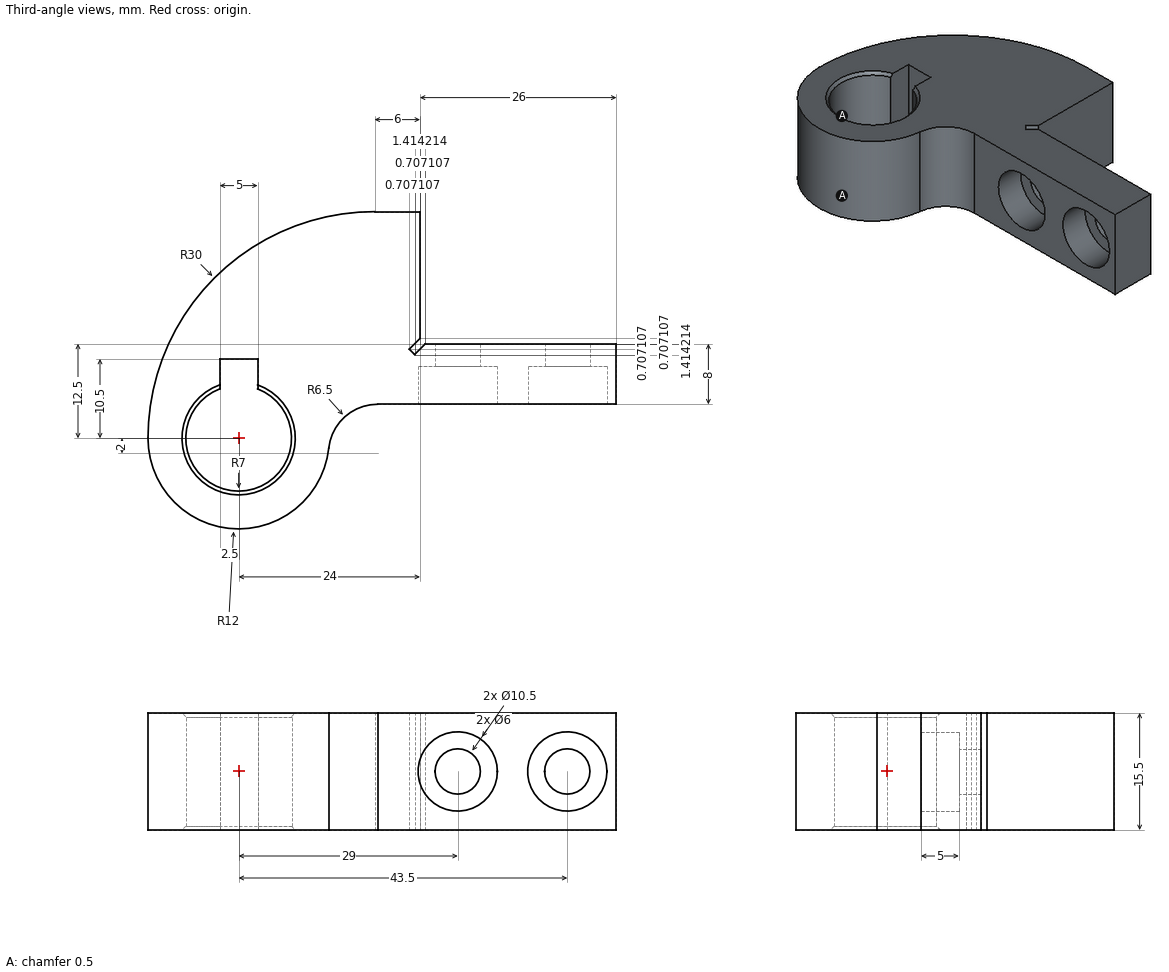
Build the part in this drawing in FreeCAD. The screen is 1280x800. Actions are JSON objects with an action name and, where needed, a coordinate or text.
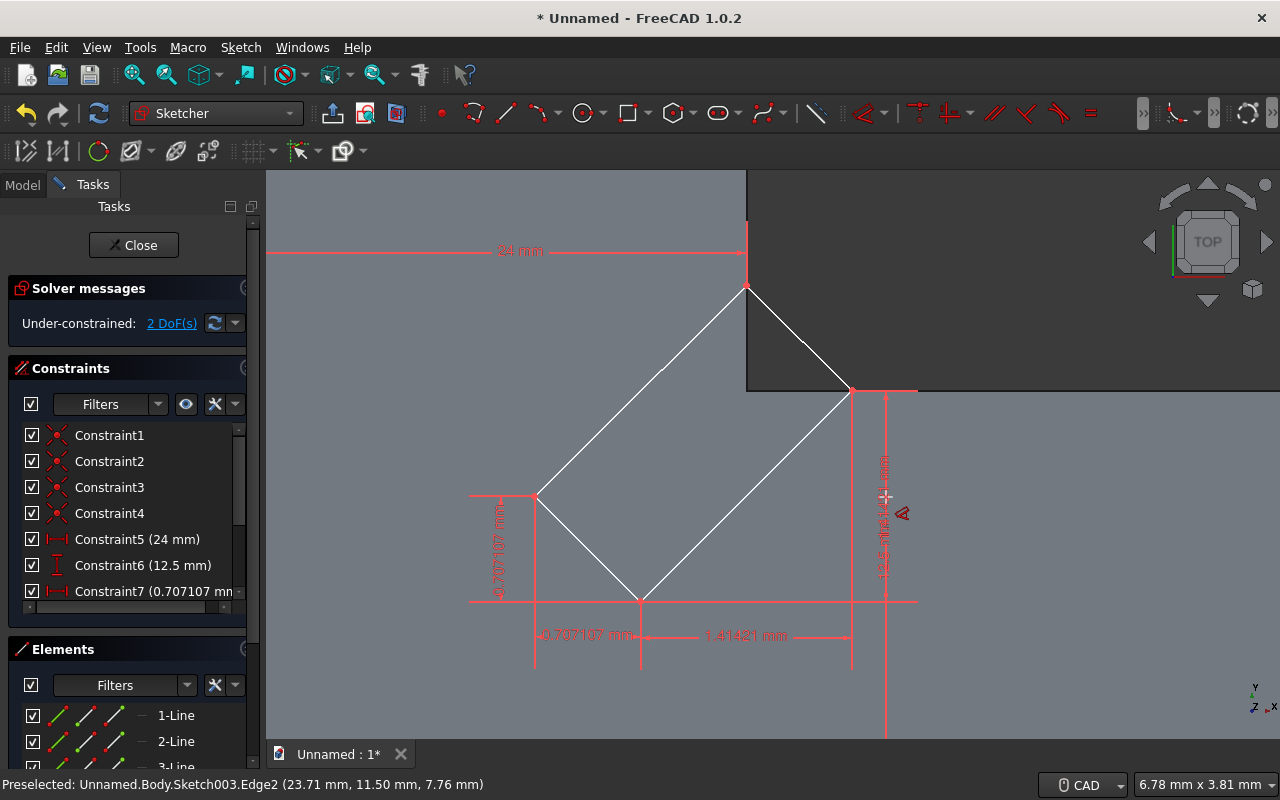
{"action": "left_click", "coordinate": [820, 359]}
{"action": "left_click", "coordinate": [799, 252]}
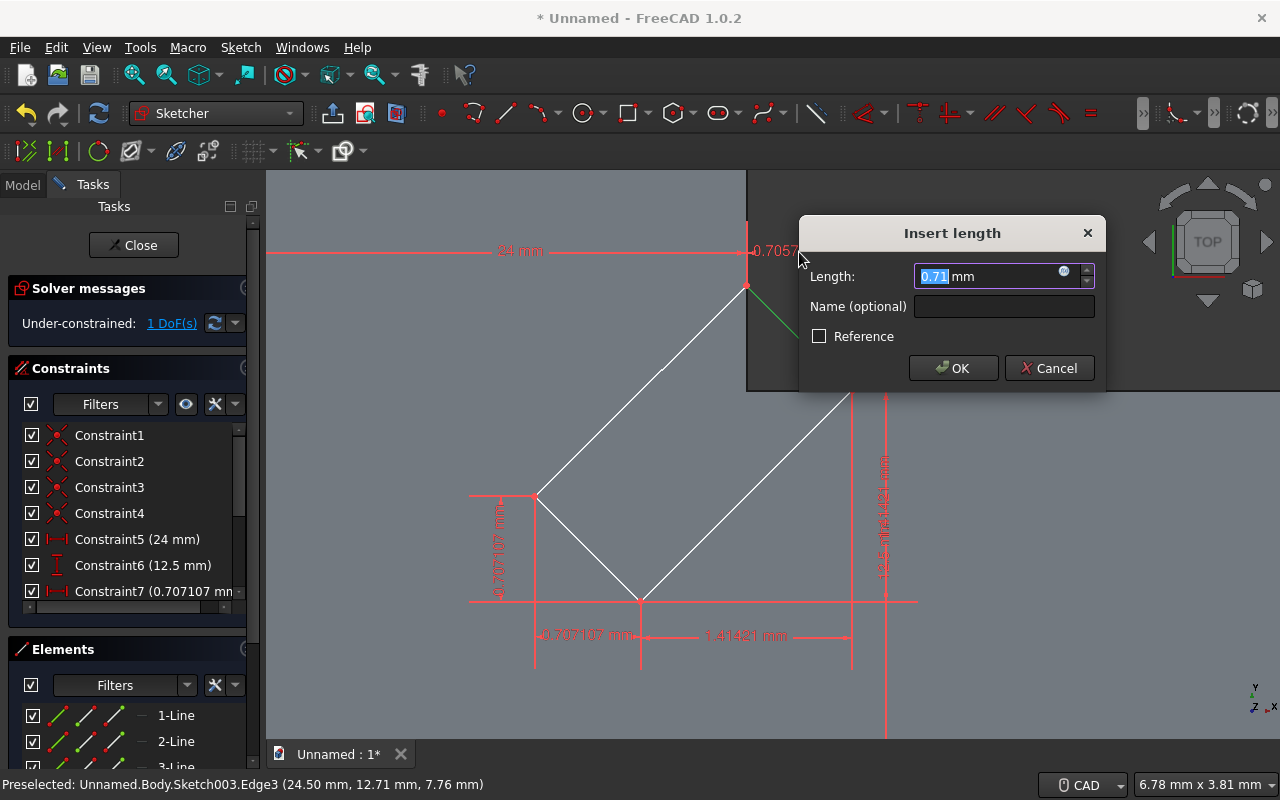
{"action": "type", "text": "0.707107"}
{"action": "key", "text": "Return"}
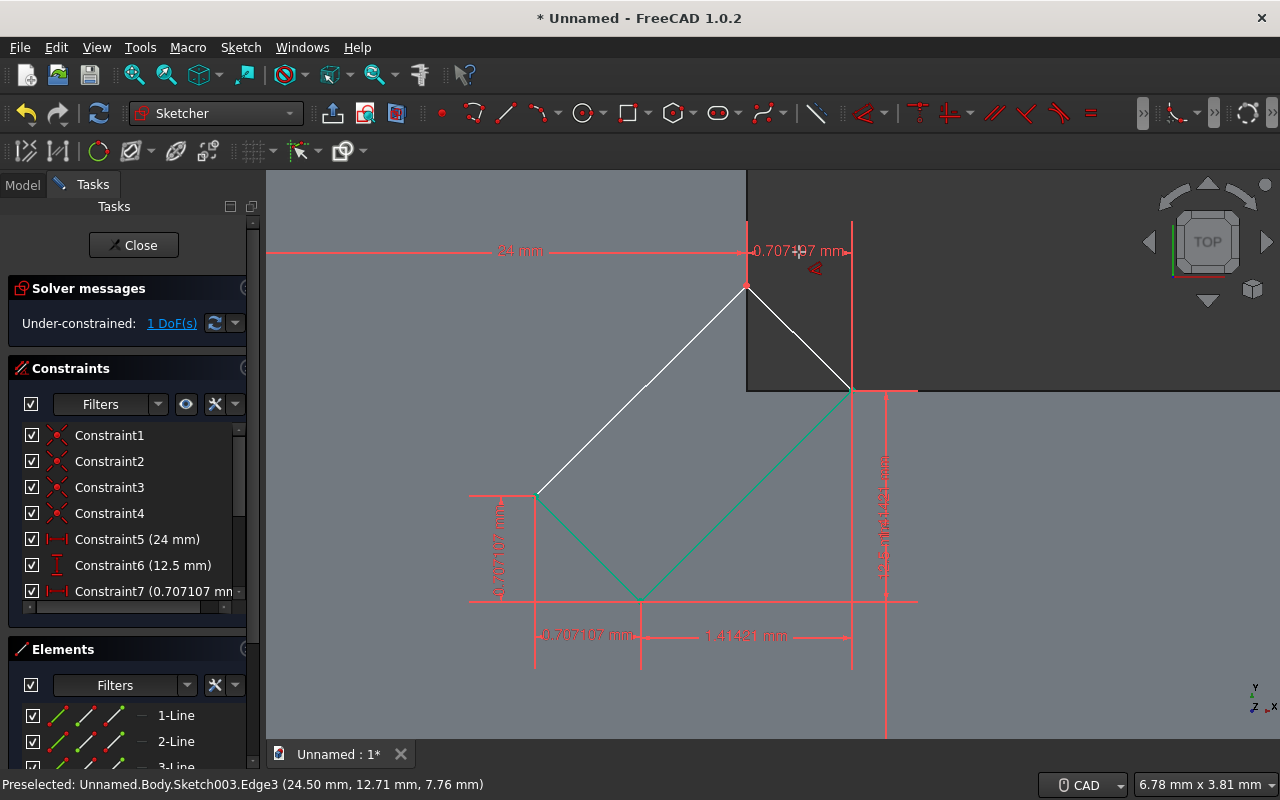
{"action": "left_click", "coordinate": [820, 359]}
{"action": "left_click", "coordinate": [886, 338]}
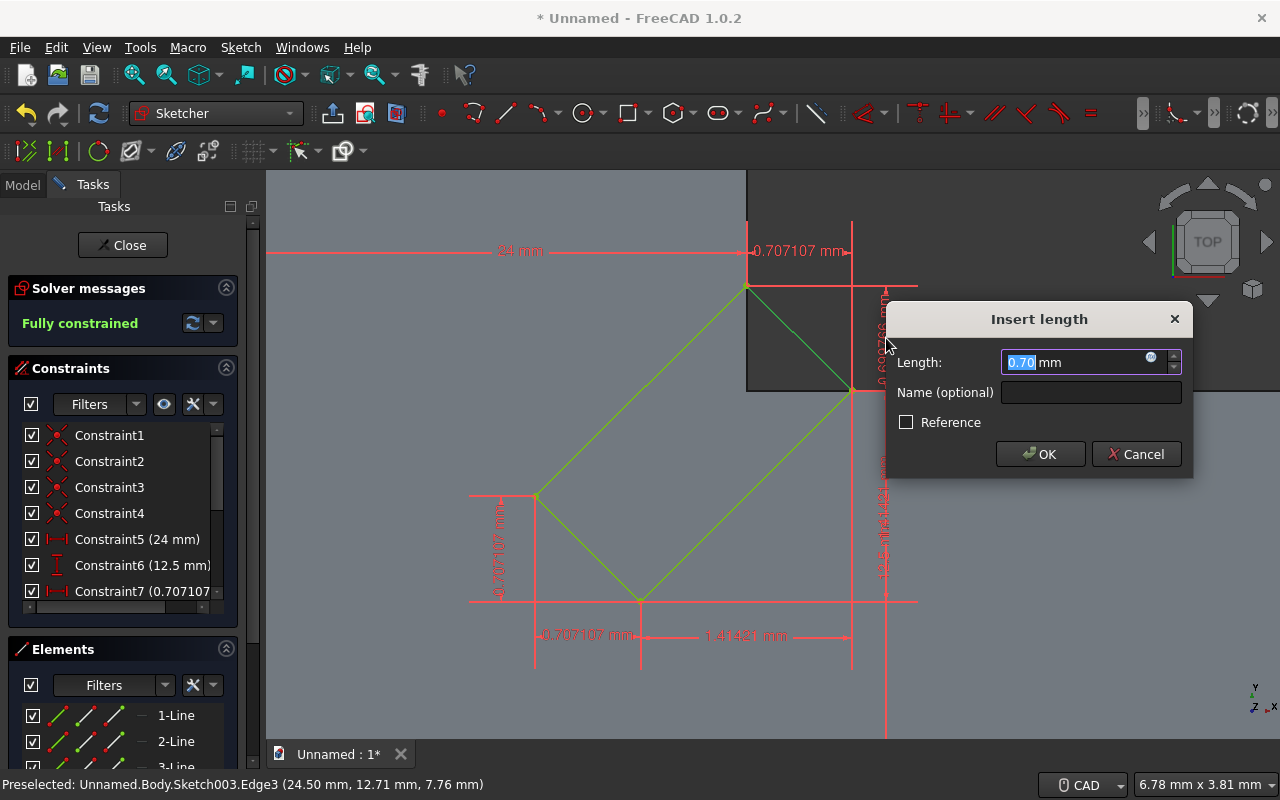
{"action": "type", "text": "0.707107"}
{"action": "key", "text": "Return"}
{"action": "key", "text": "Escape"}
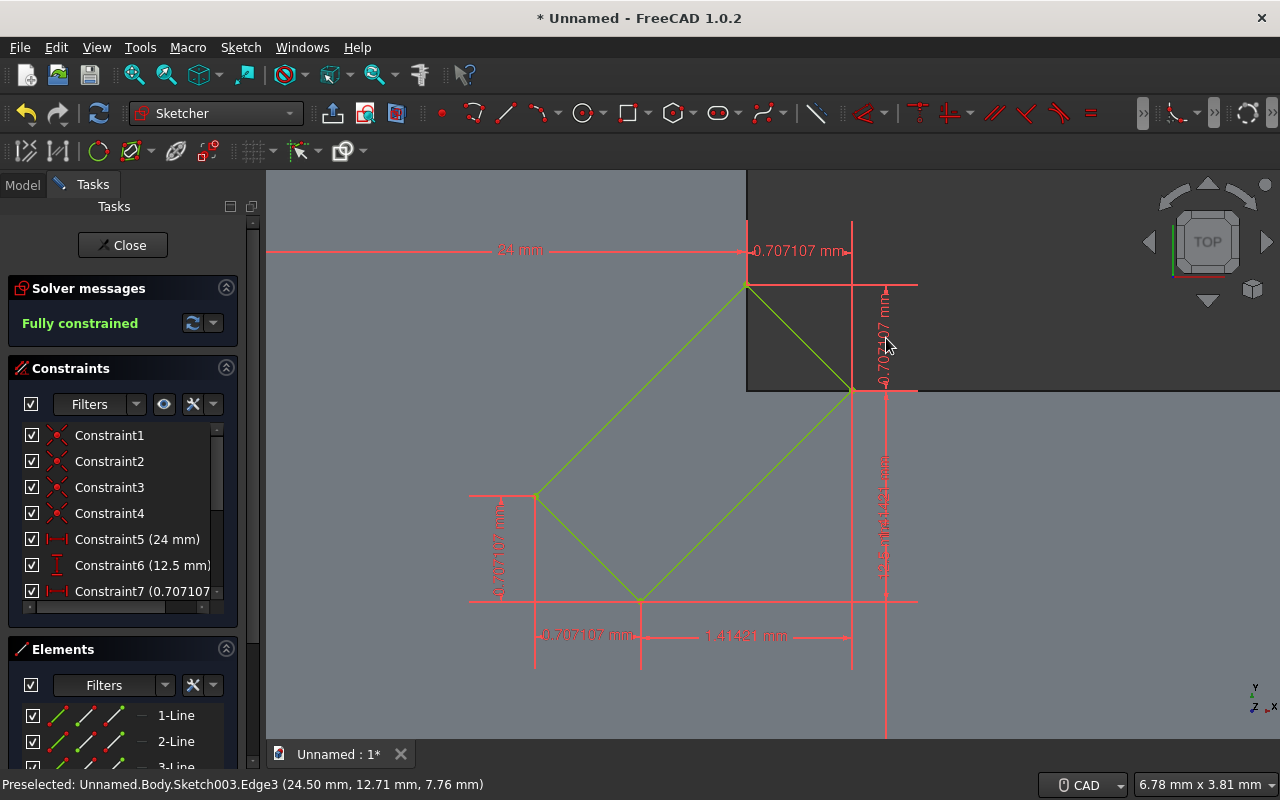
{"action": "left_click", "coordinate": [123, 245]}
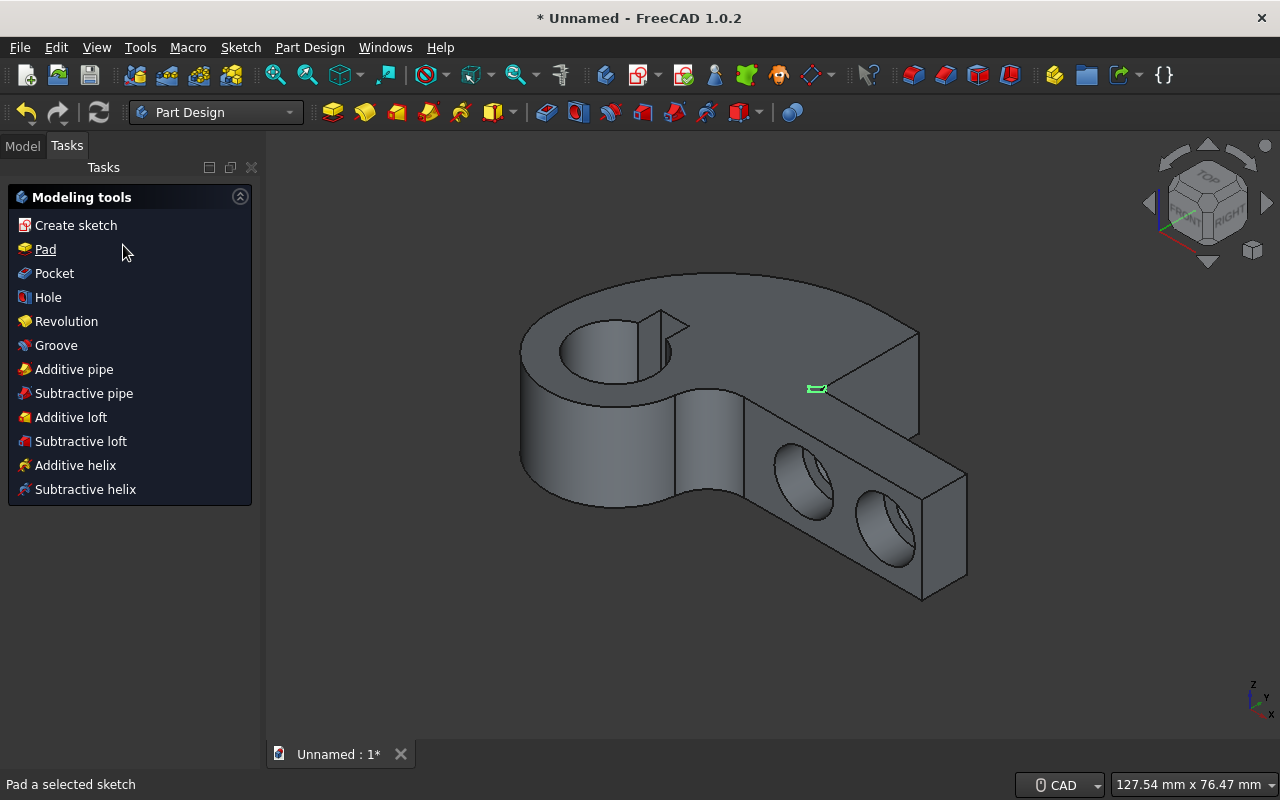
{"action": "left_click", "coordinate": [548, 112]}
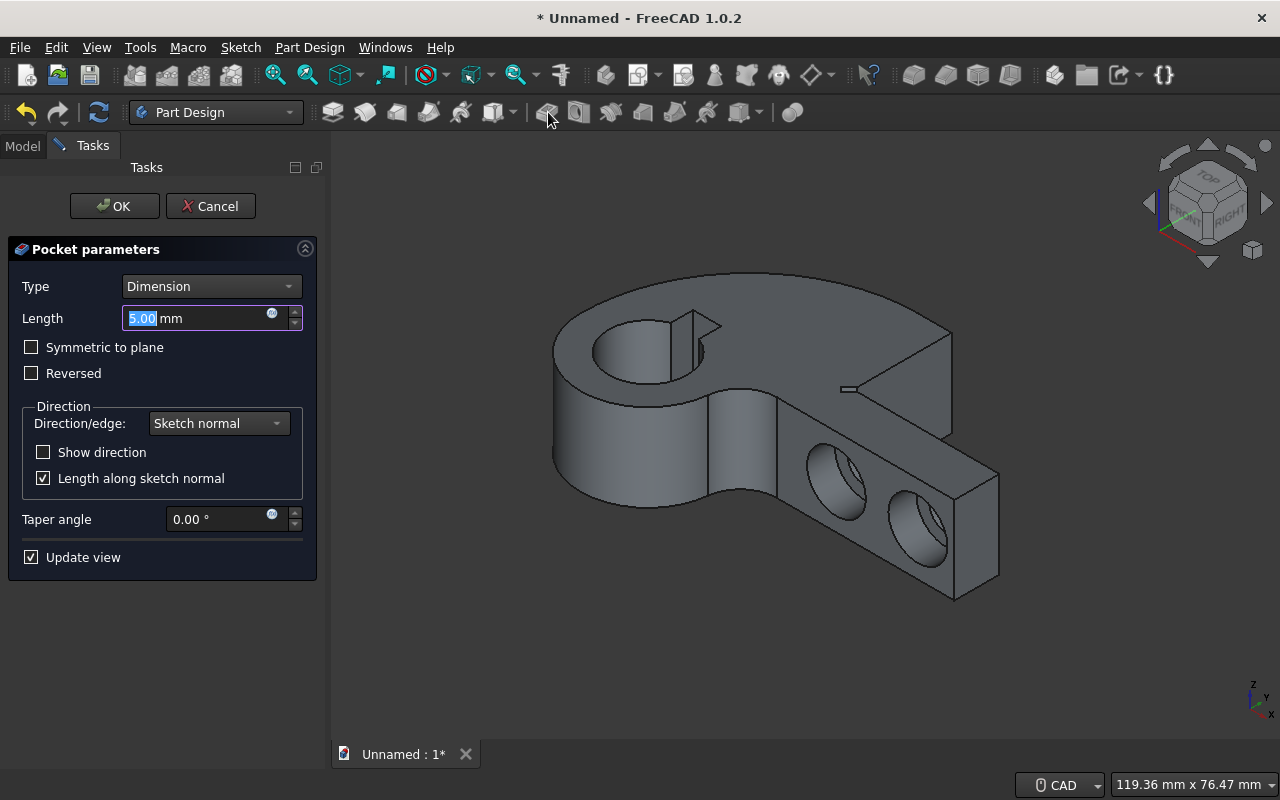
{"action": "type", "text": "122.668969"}
{"action": "key", "text": "Tab"}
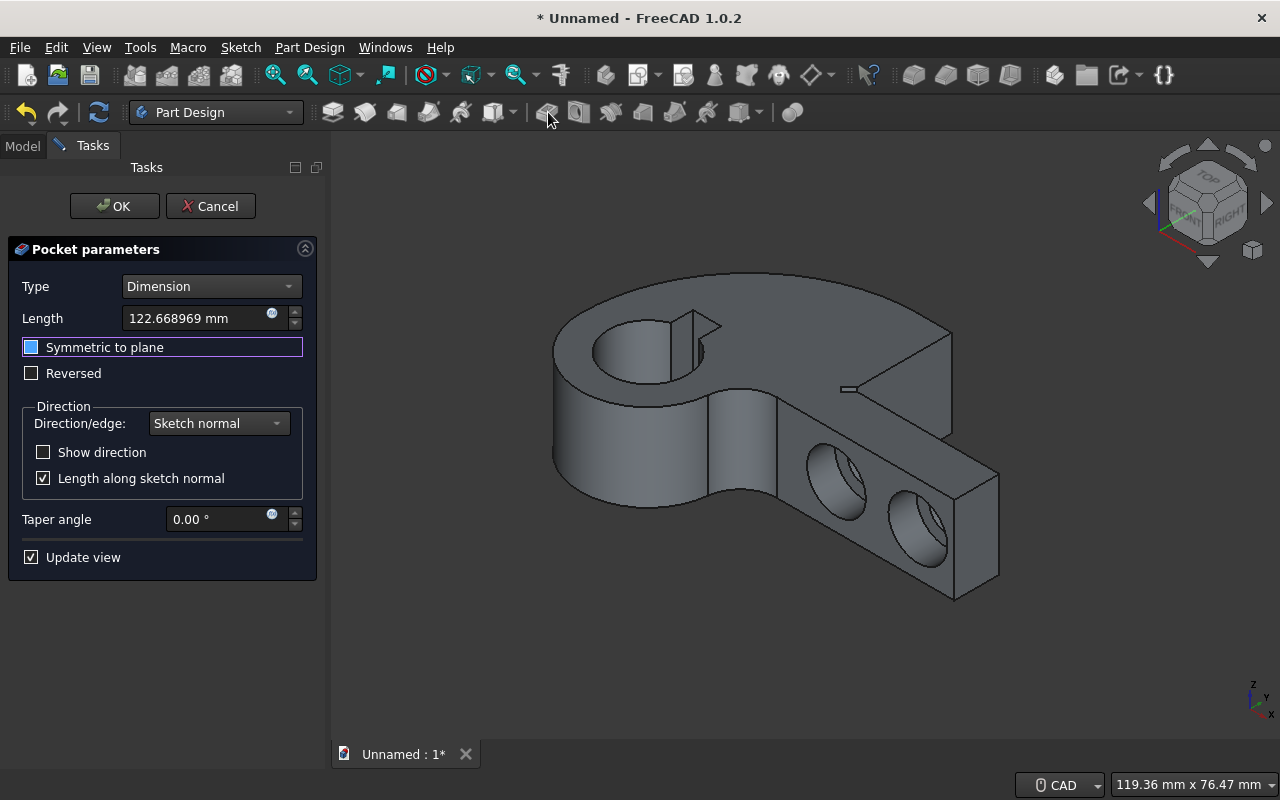
{"action": "left_click", "coordinate": [30, 347]}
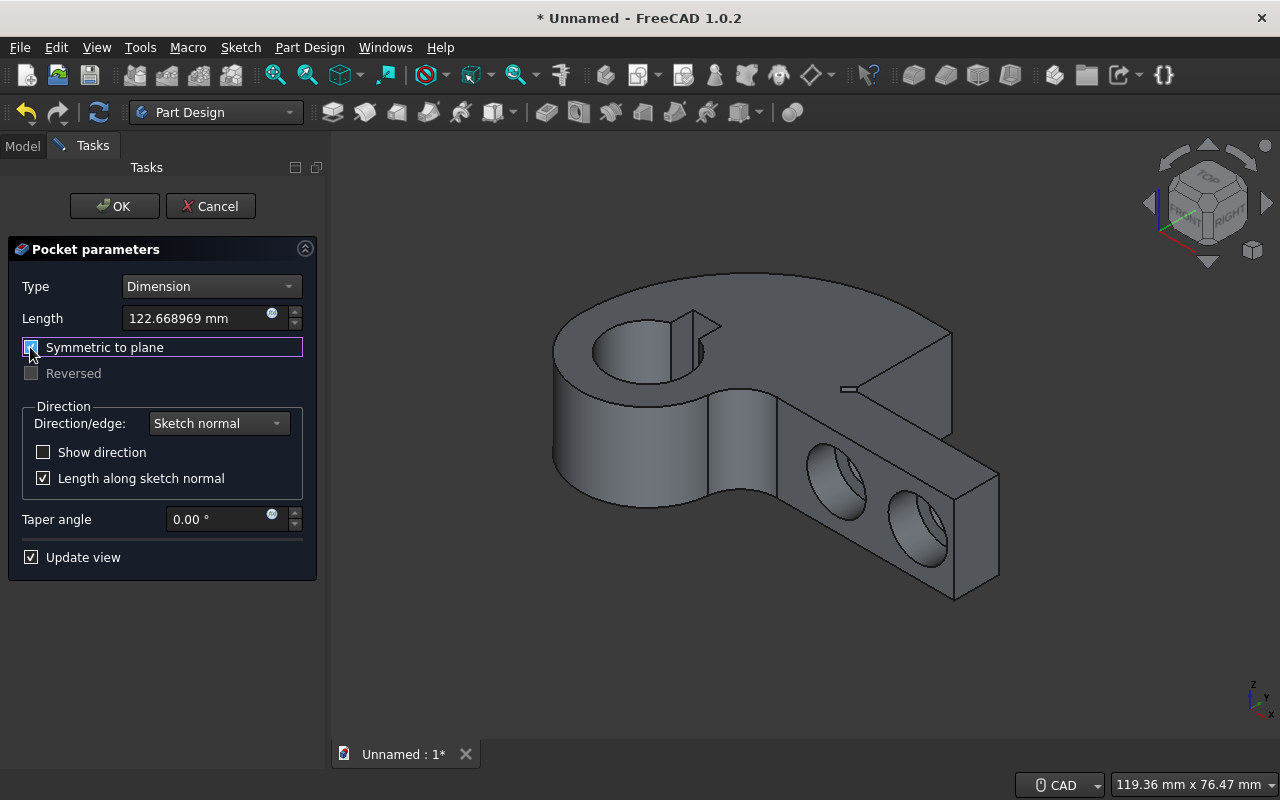
{"action": "left_click", "coordinate": [115, 206]}